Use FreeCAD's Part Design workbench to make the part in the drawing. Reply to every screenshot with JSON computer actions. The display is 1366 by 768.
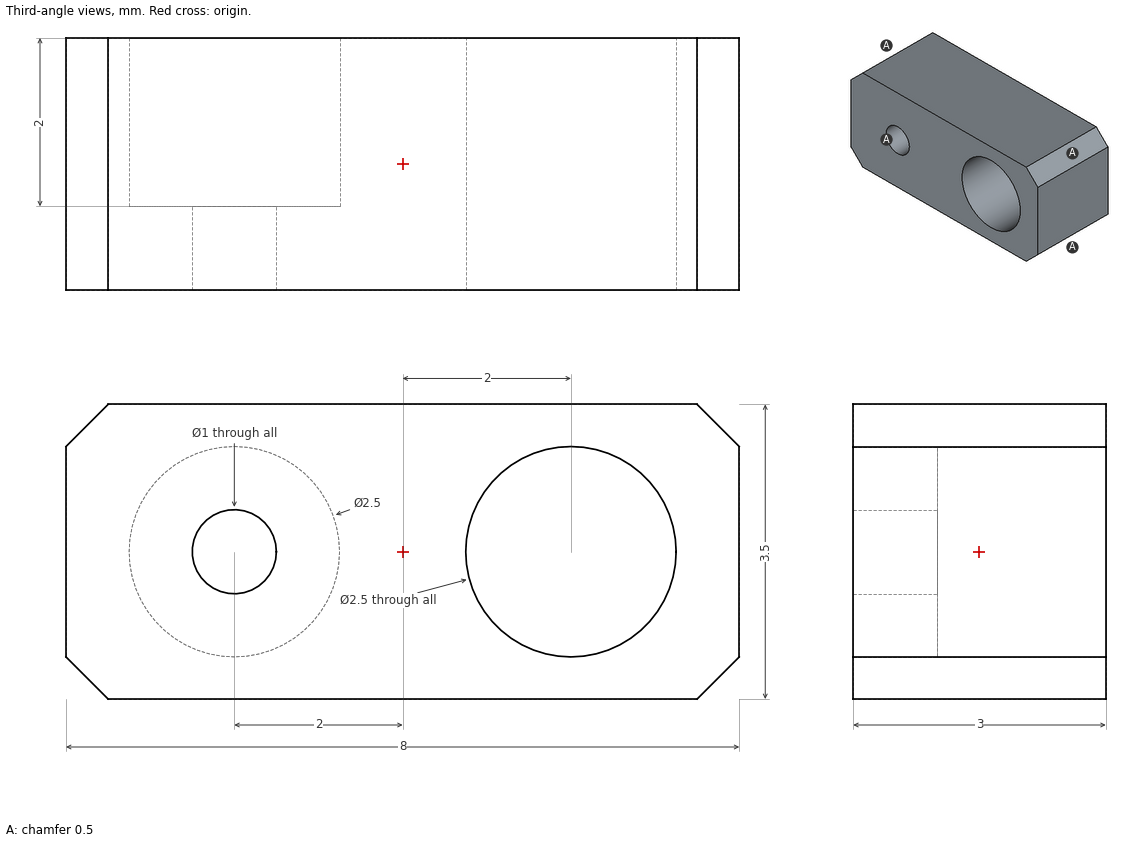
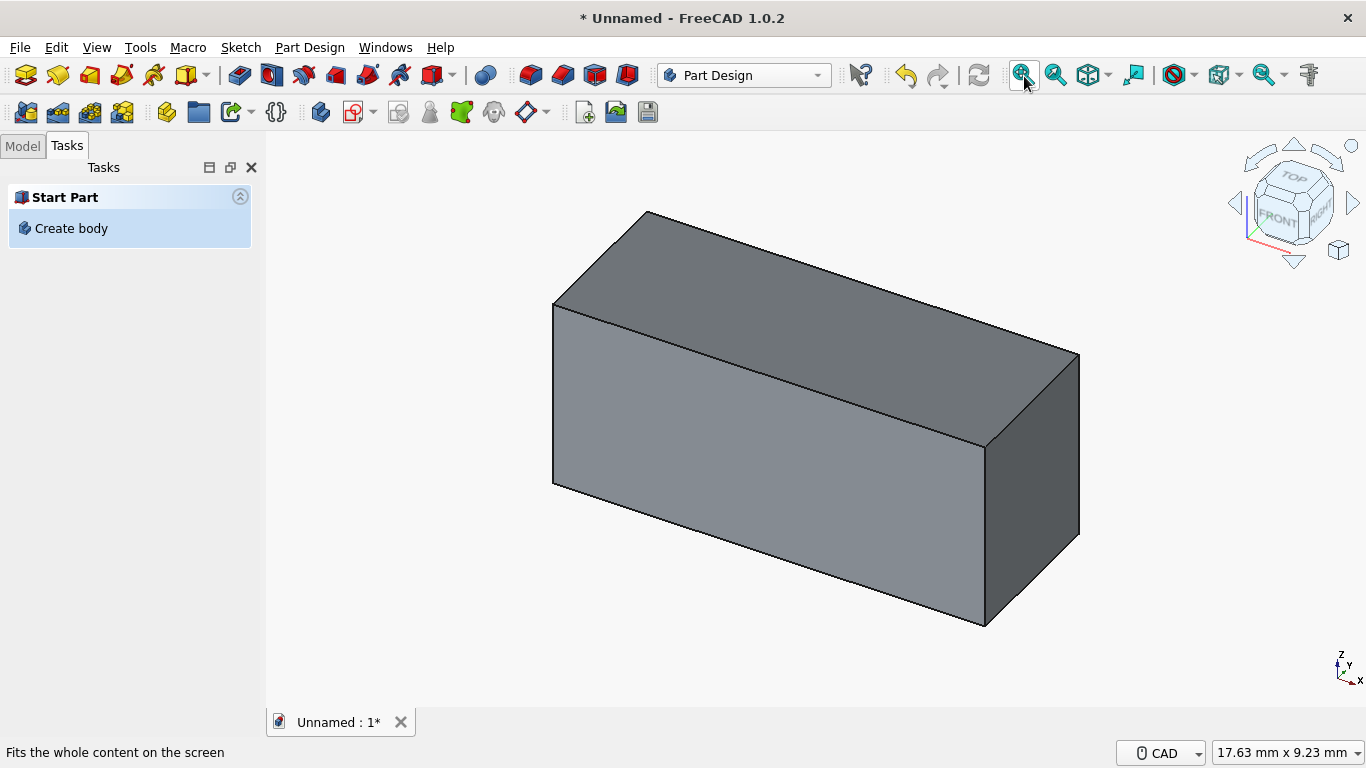
{"action": "key", "text": "4"}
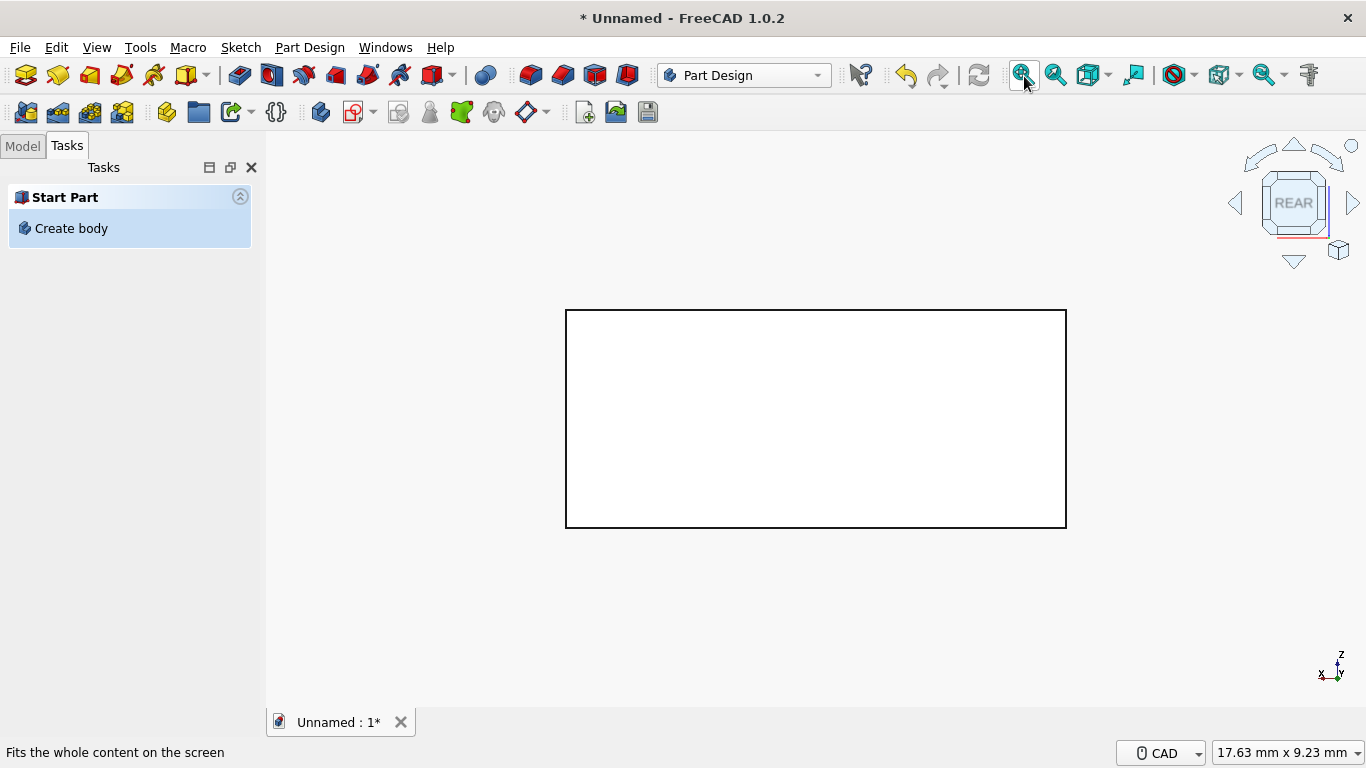
{"action": "left_click", "coordinate": [745, 418]}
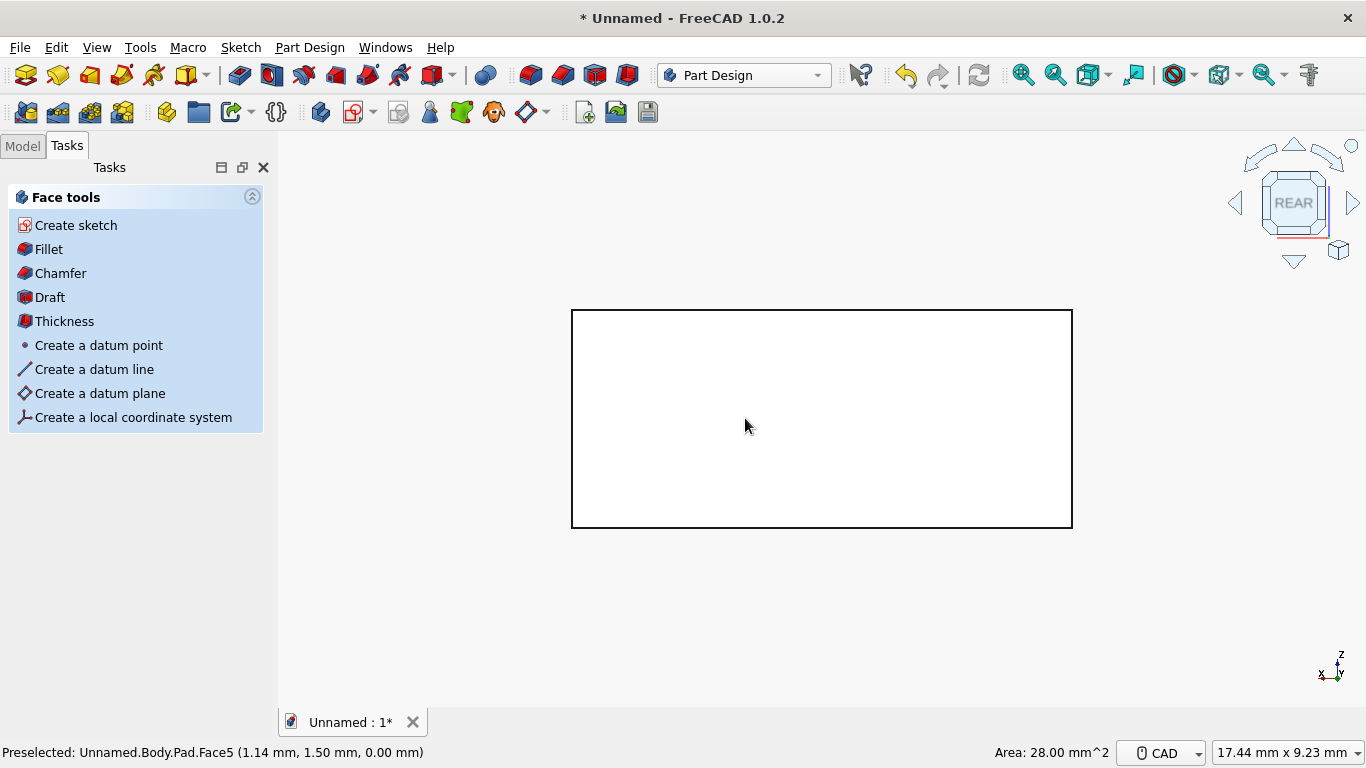
{"action": "left_click", "coordinate": [354, 112]}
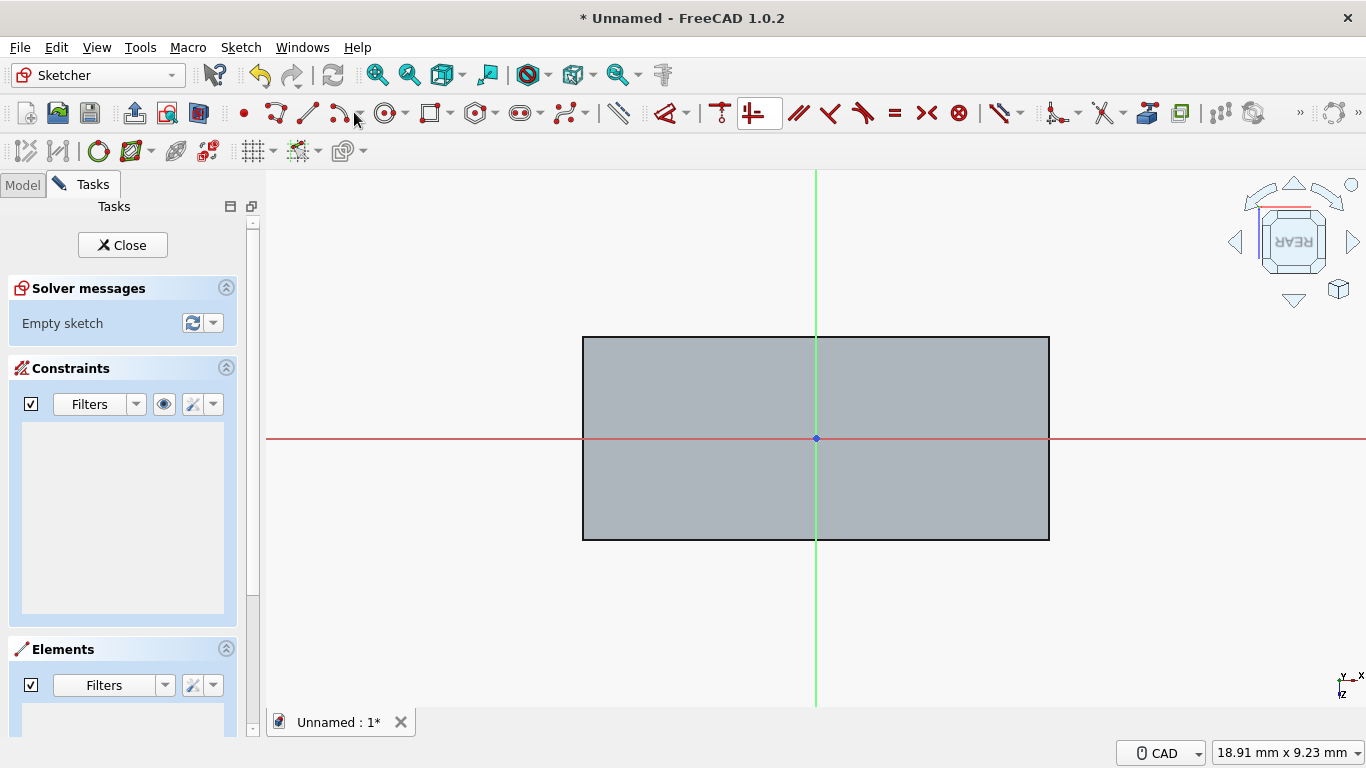
{"action": "scroll", "coordinate": [700, 439], "scroll_direction": "up", "scroll_amount": 4}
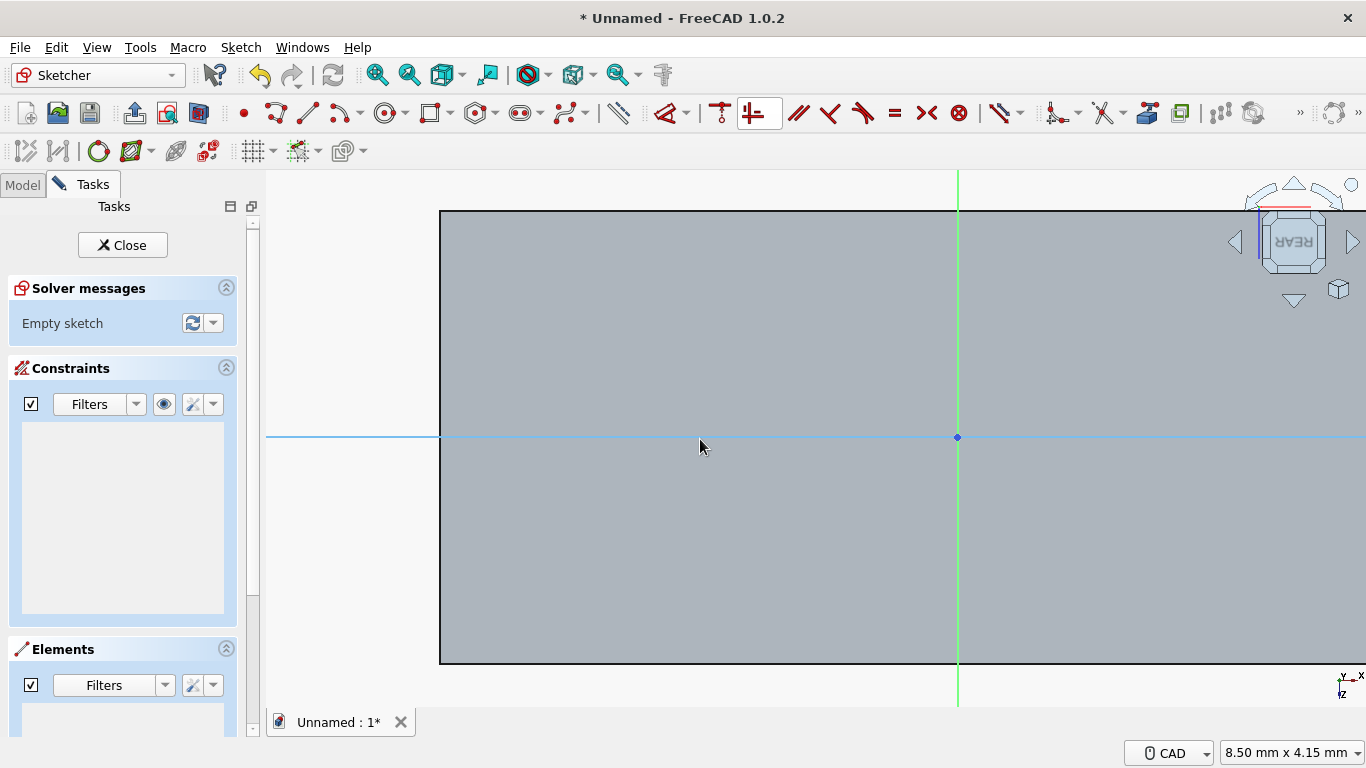
{"action": "left_click", "coordinate": [386, 114]}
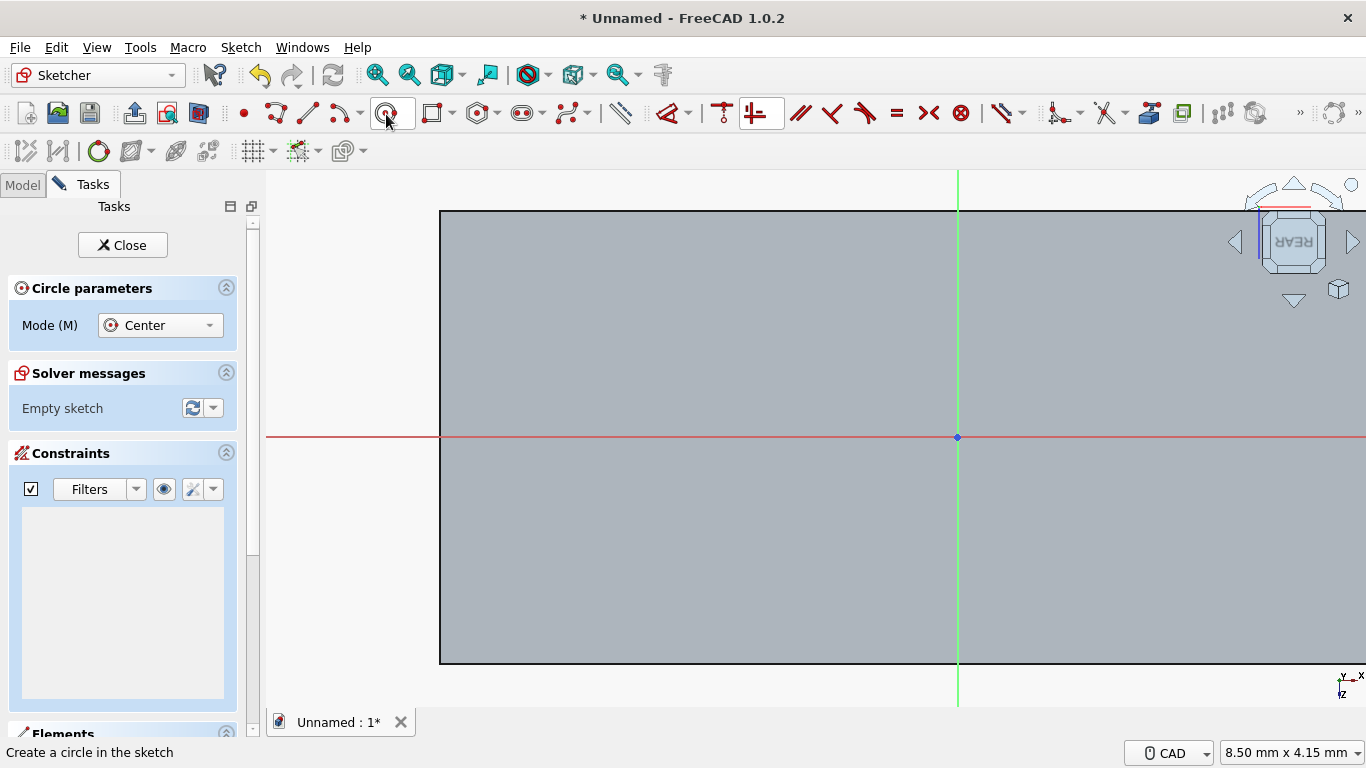
{"action": "left_click", "coordinate": [699, 437]}
{"action": "left_click", "coordinate": [813, 323]}
{"action": "key", "text": "Escape"}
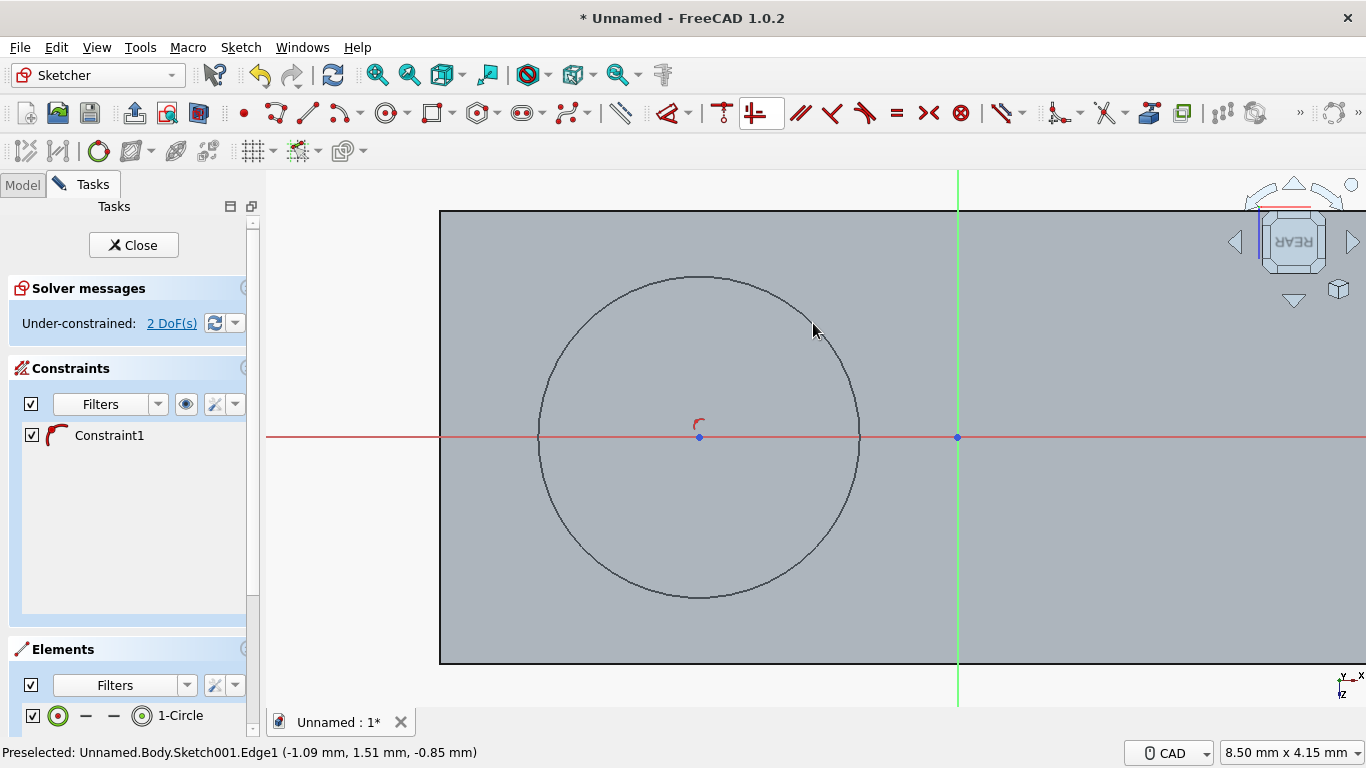
{"action": "left_click", "coordinate": [668, 114]}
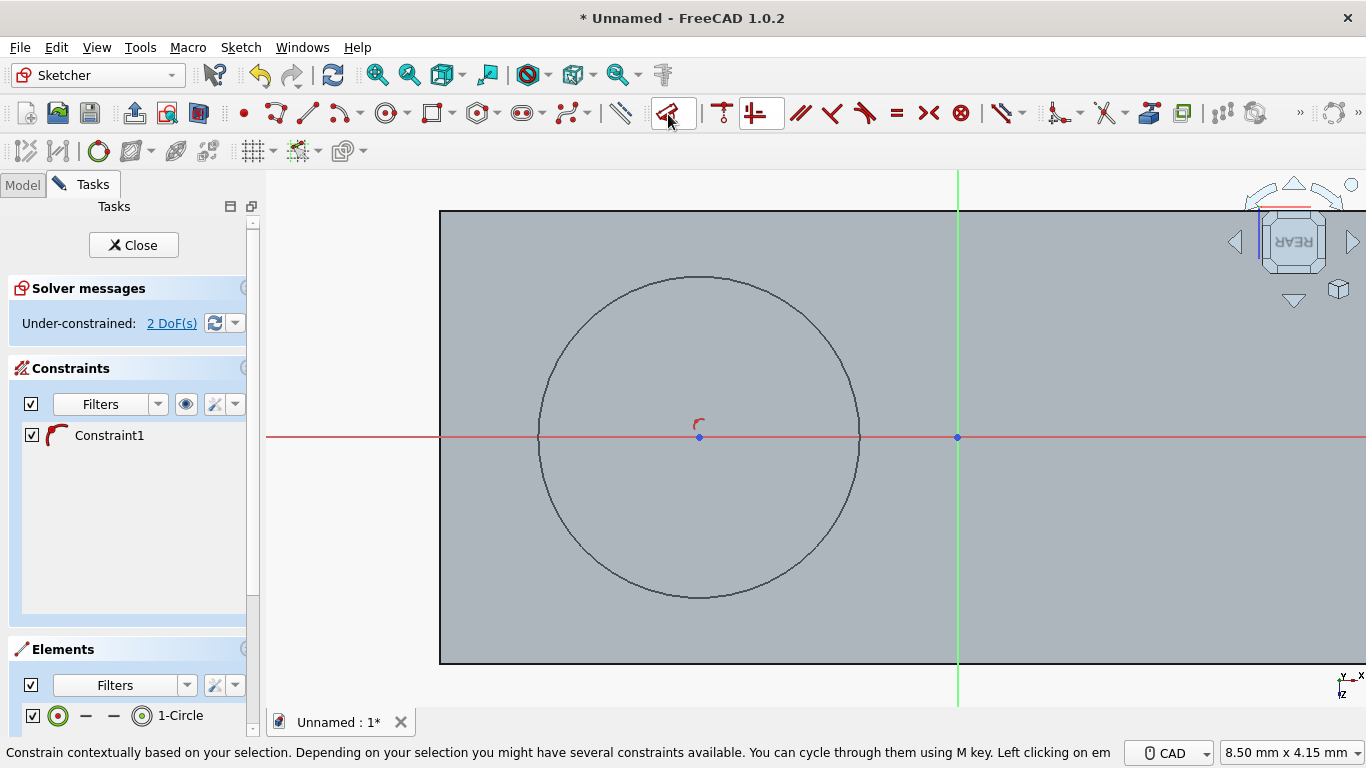
{"action": "left_click", "coordinate": [812, 323]}
{"action": "left_click", "coordinate": [835, 300]}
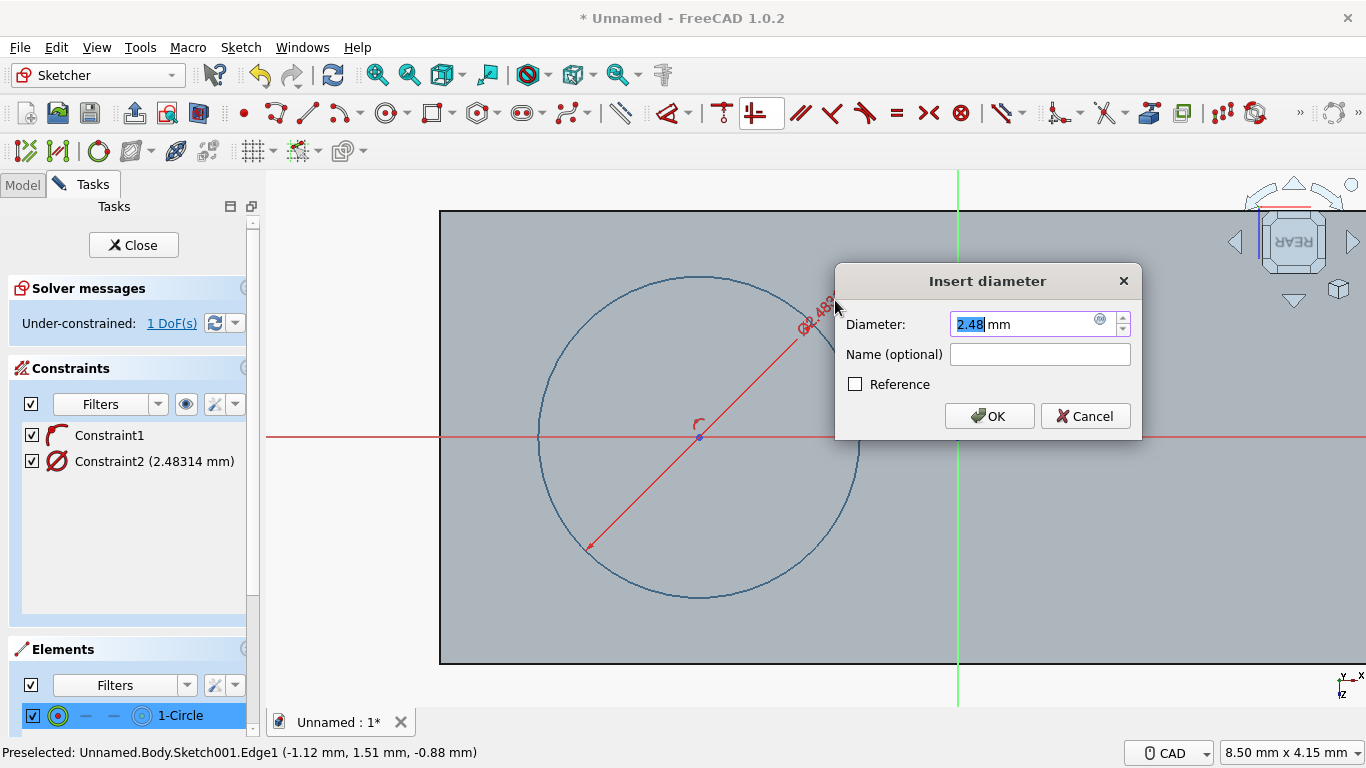
{"action": "type", "text": "2.5"}
{"action": "key", "text": "Return"}